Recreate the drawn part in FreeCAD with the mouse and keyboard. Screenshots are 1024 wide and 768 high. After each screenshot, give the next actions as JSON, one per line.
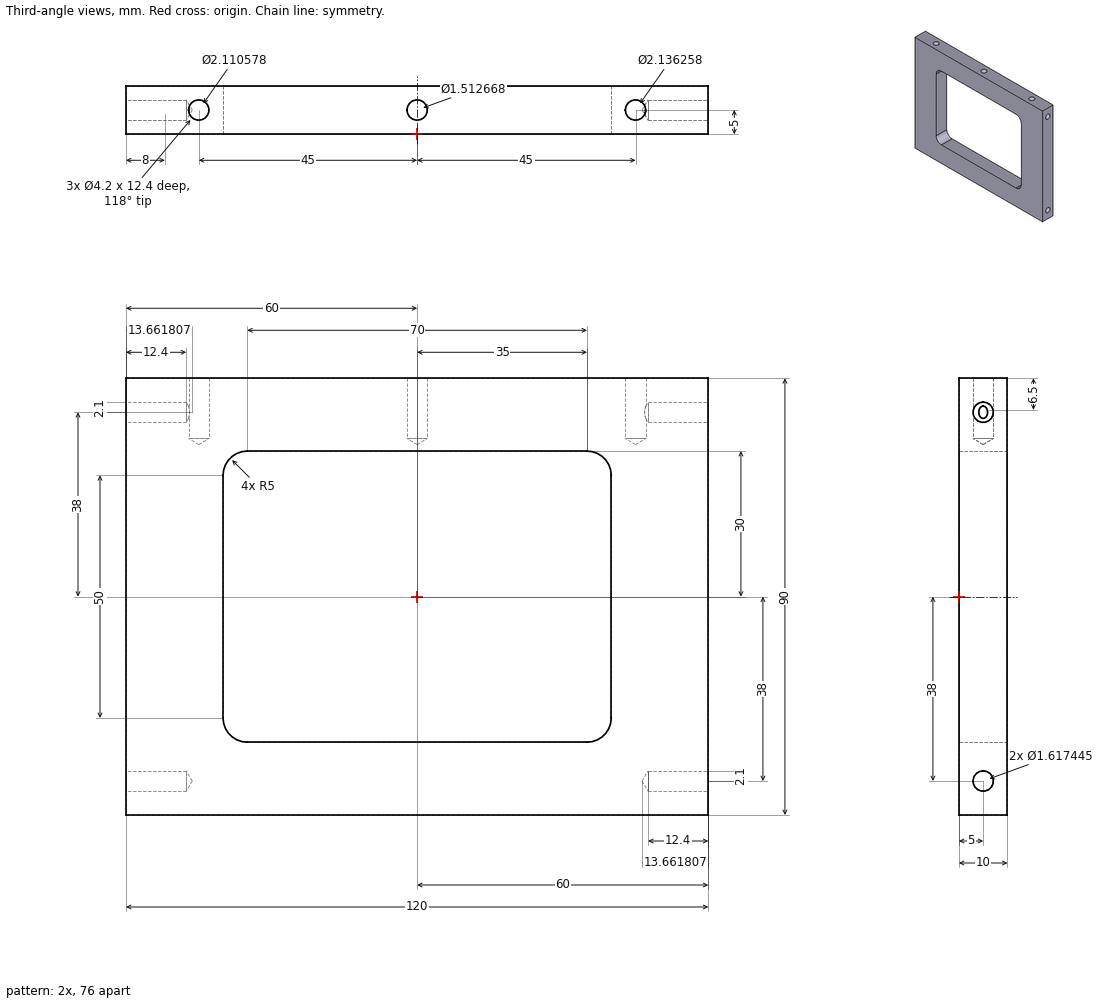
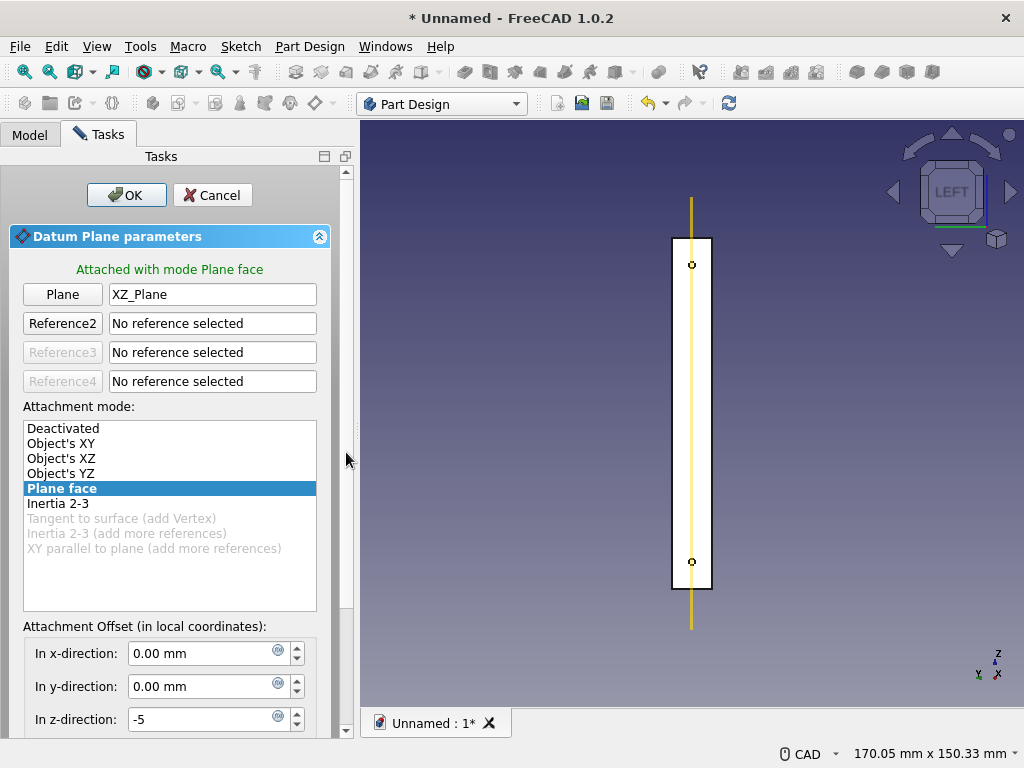
{"action": "left_click", "coordinate": [127, 195]}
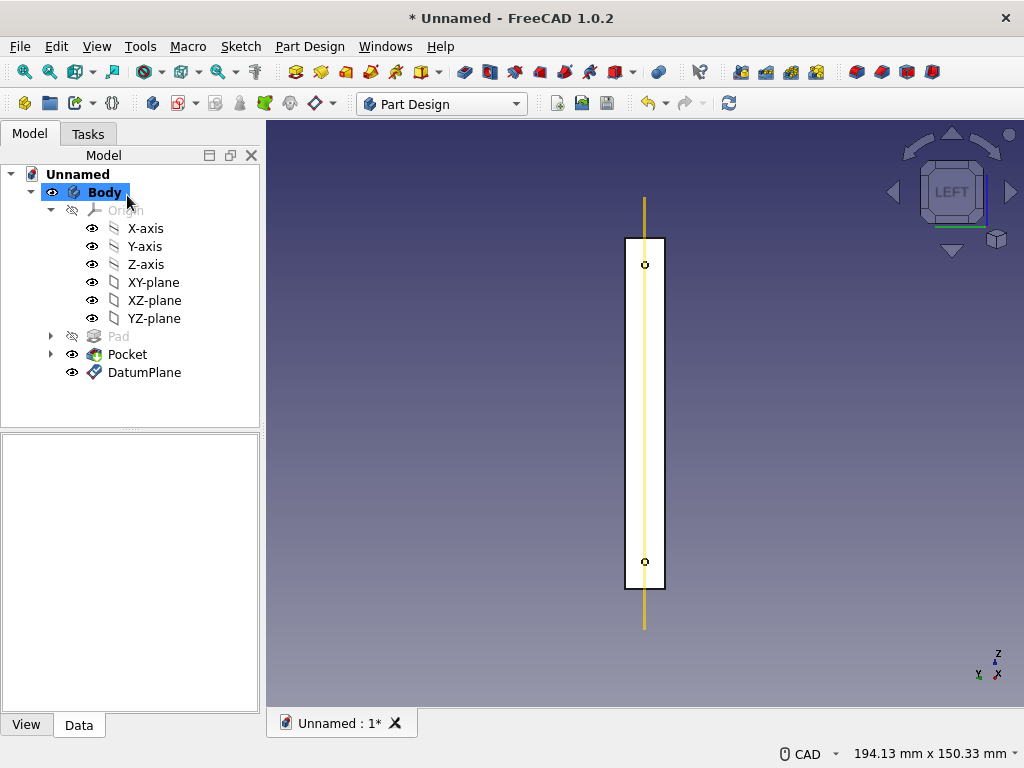
{"action": "left_click", "coordinate": [117, 372]}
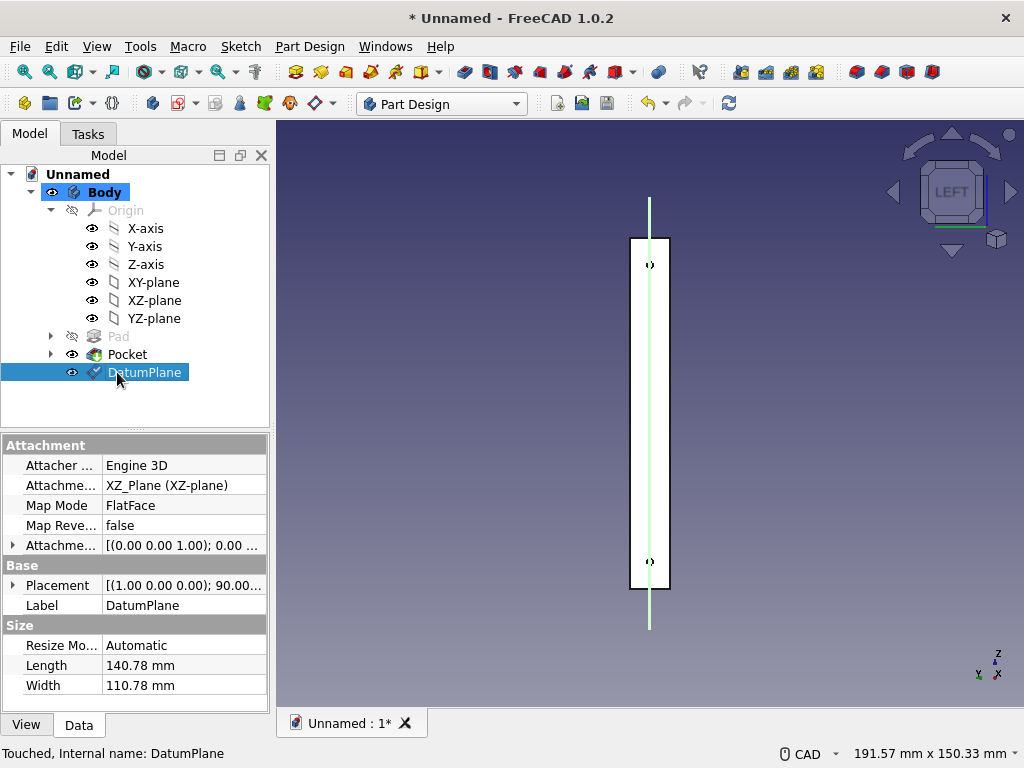
{"action": "left_click", "coordinate": [178, 104]}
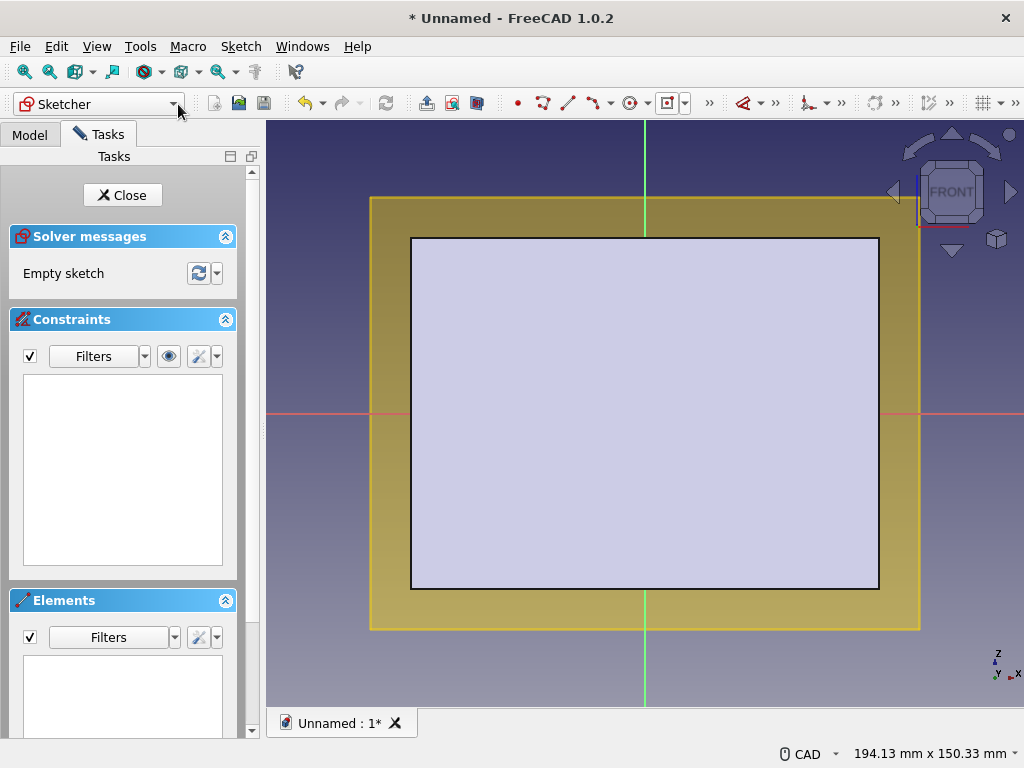
{"action": "left_click", "coordinate": [477, 104]}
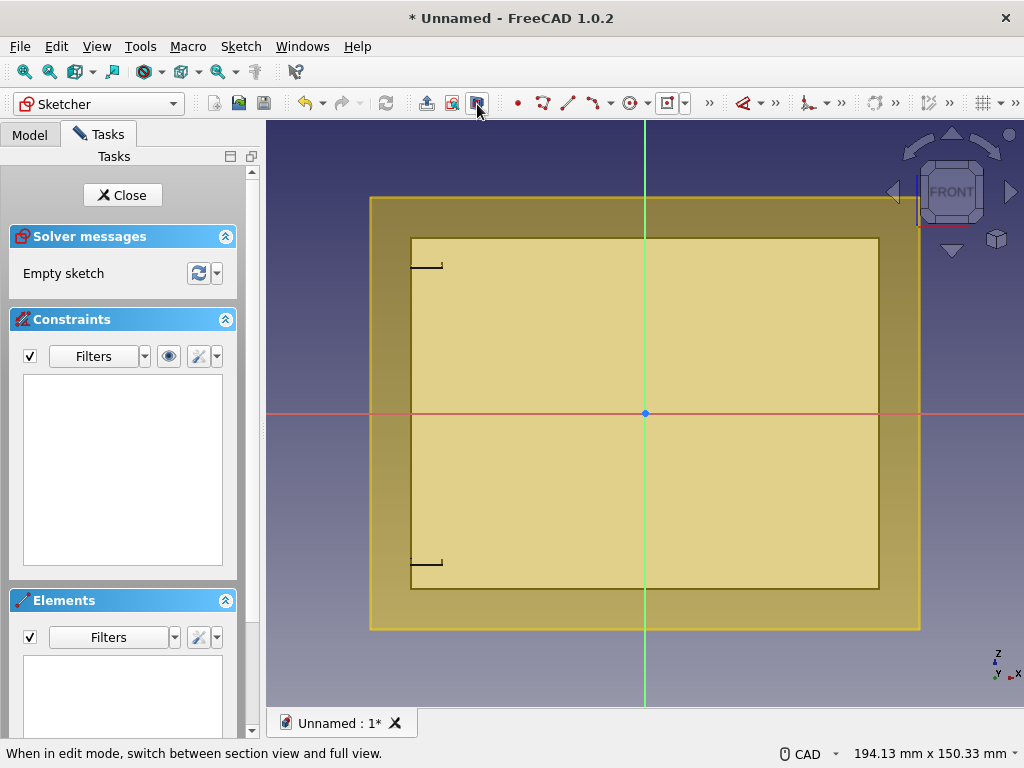
{"action": "scroll", "coordinate": [416, 222], "scroll_direction": "up", "scroll_amount": 8}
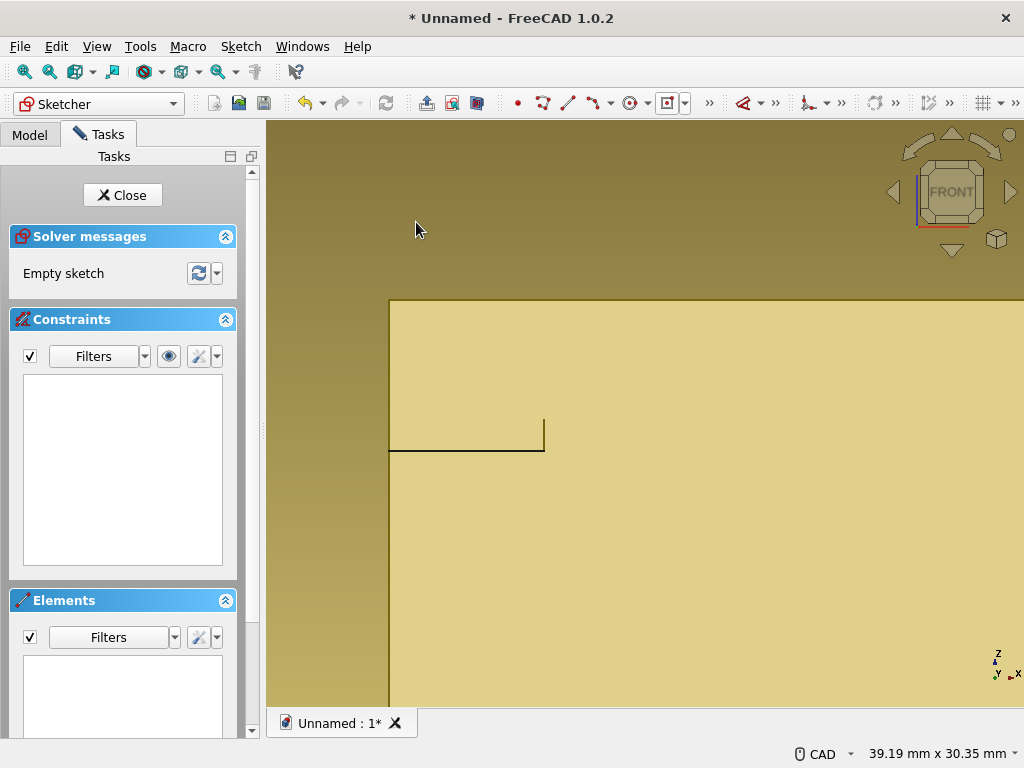
{"action": "left_click", "coordinate": [543, 104]}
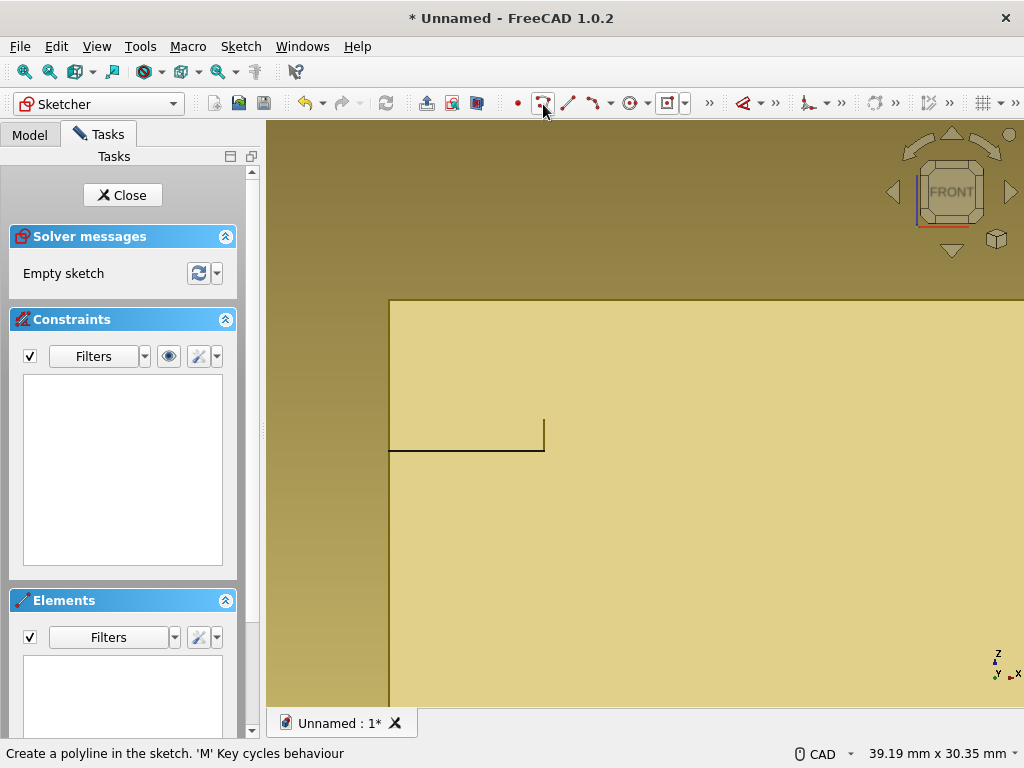
{"action": "left_click", "coordinate": [653, 435]}
{"action": "left_click", "coordinate": [389, 435]}
{"action": "left_click", "coordinate": [389, 394]}
{"action": "left_click", "coordinate": [629, 394]}
{"action": "left_click", "coordinate": [653, 436]}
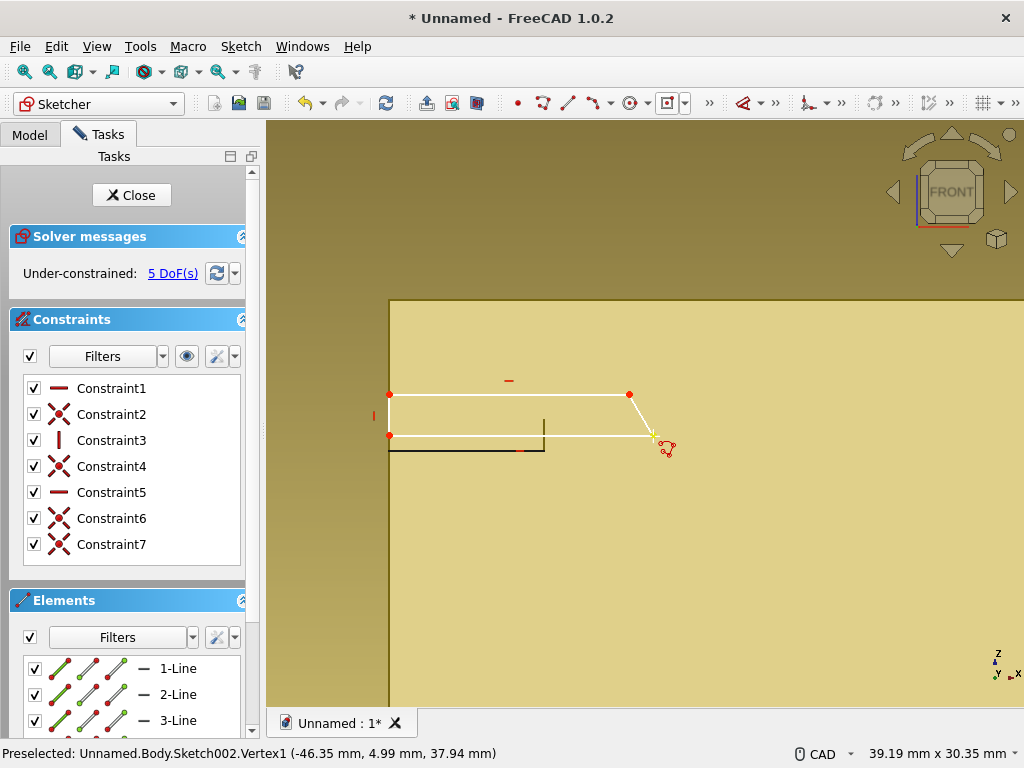
{"action": "left_click", "coordinate": [568, 104]}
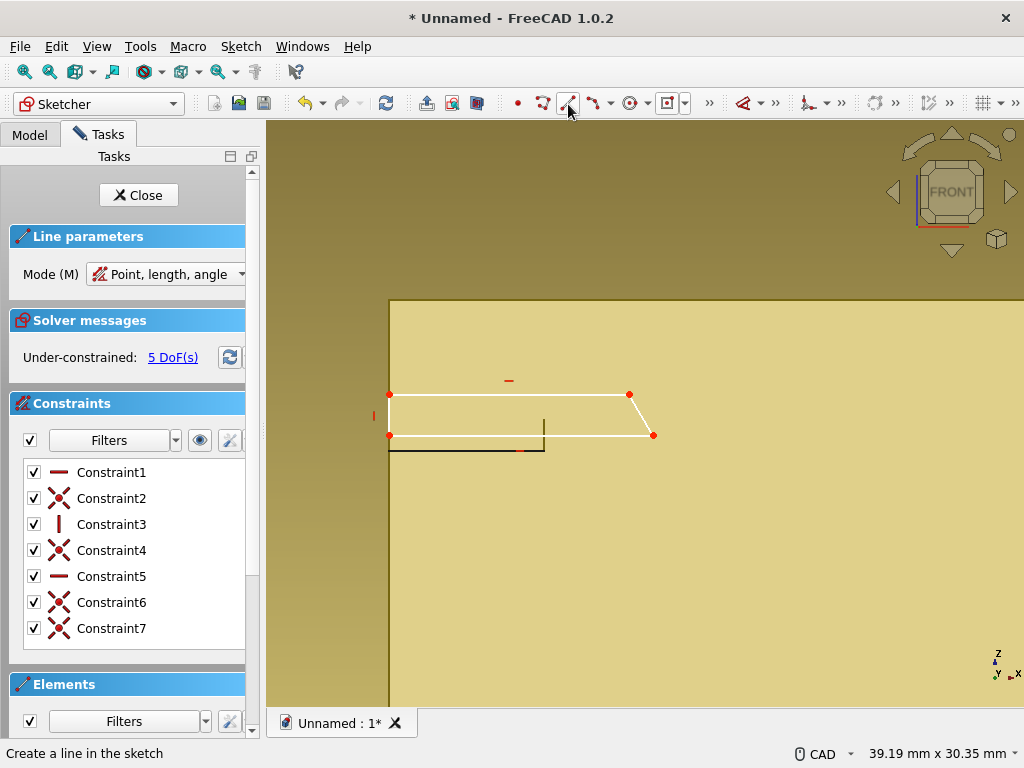
{"action": "left_click", "coordinate": [680, 435]}
{"action": "left_click", "coordinate": [759, 435]}
{"action": "key", "text": "Escape"}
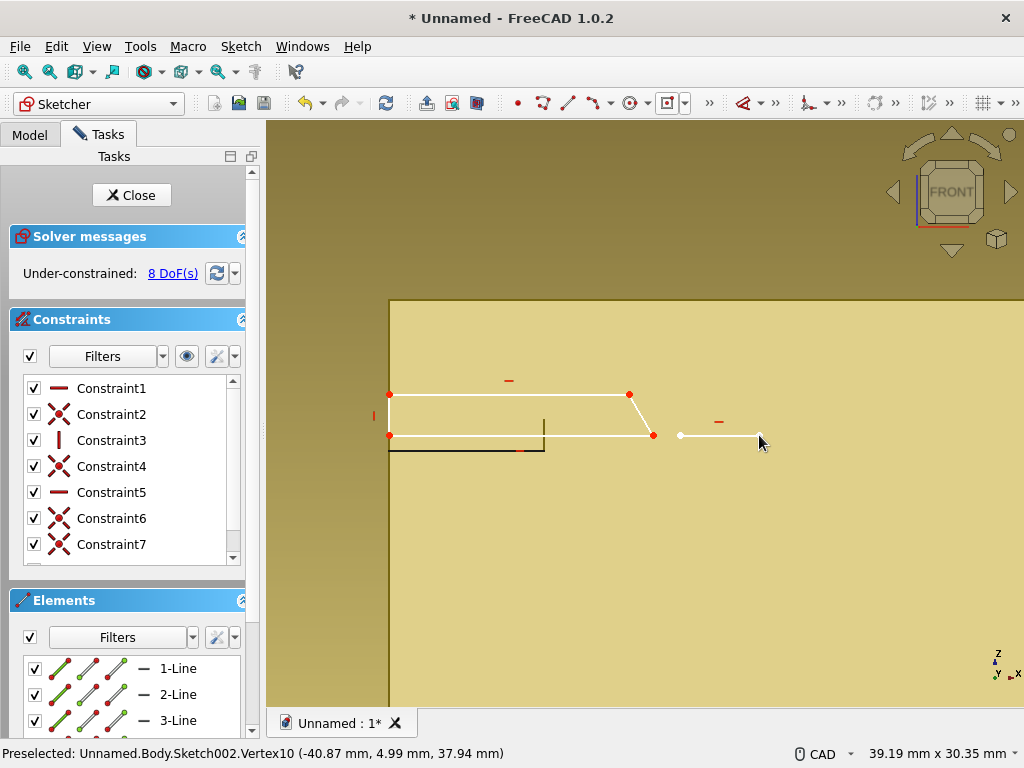
{"action": "left_click", "coordinate": [704, 436]}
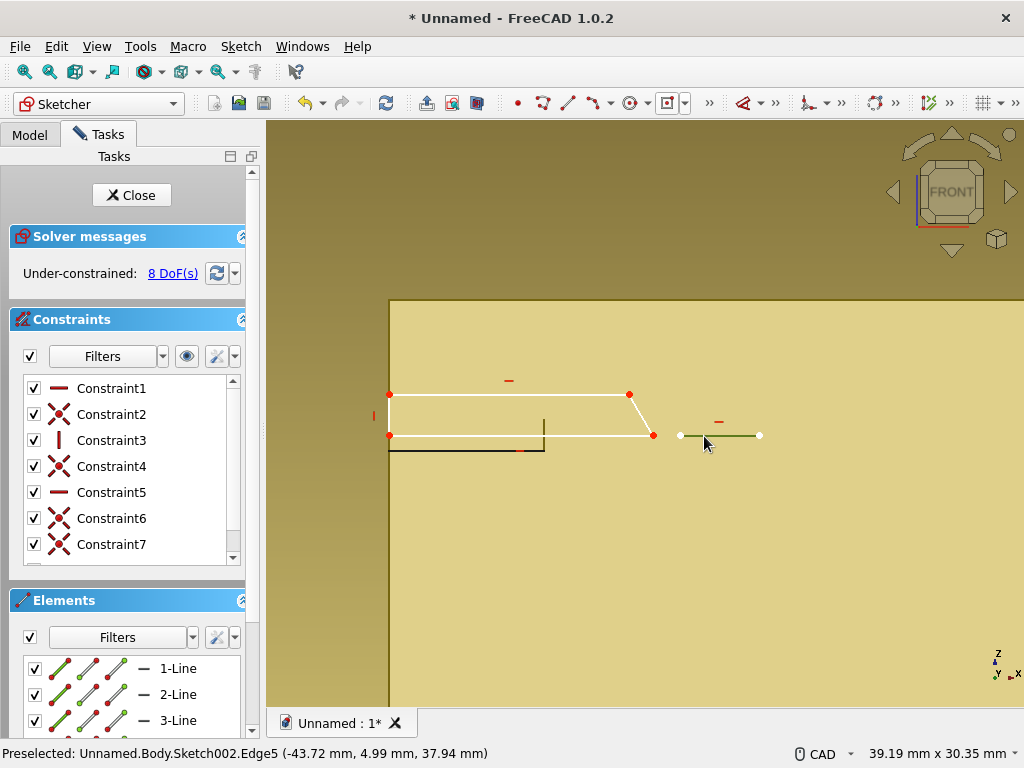
{"action": "key", "text": "g n"}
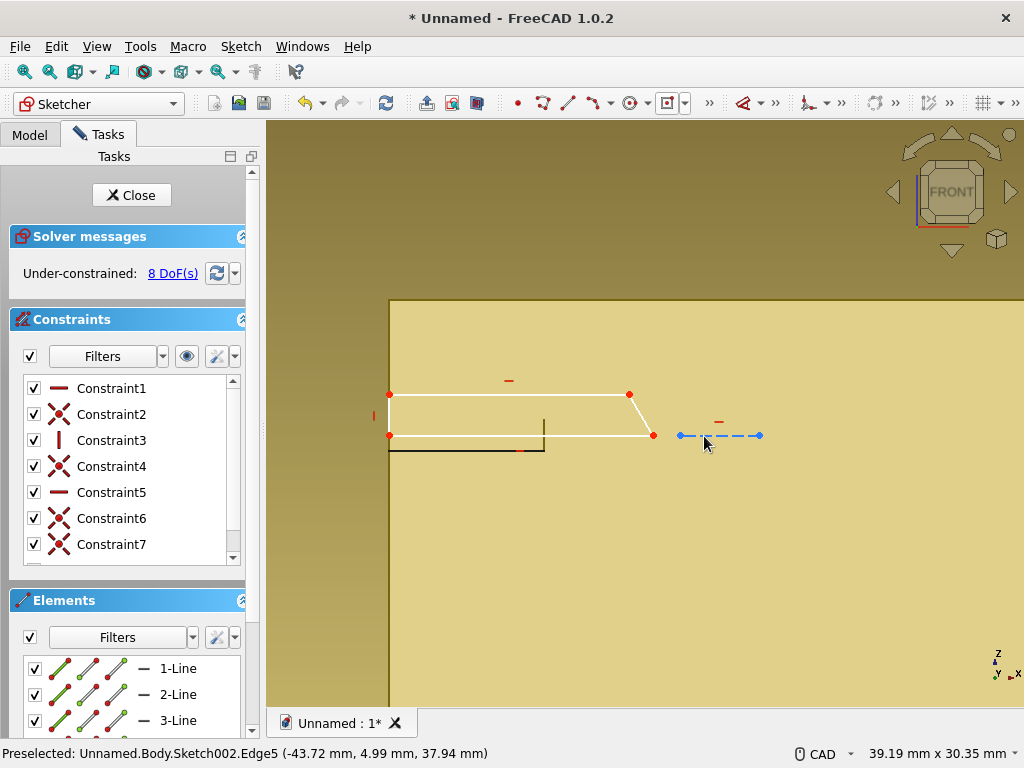
{"action": "left_click", "coordinate": [742, 104]}